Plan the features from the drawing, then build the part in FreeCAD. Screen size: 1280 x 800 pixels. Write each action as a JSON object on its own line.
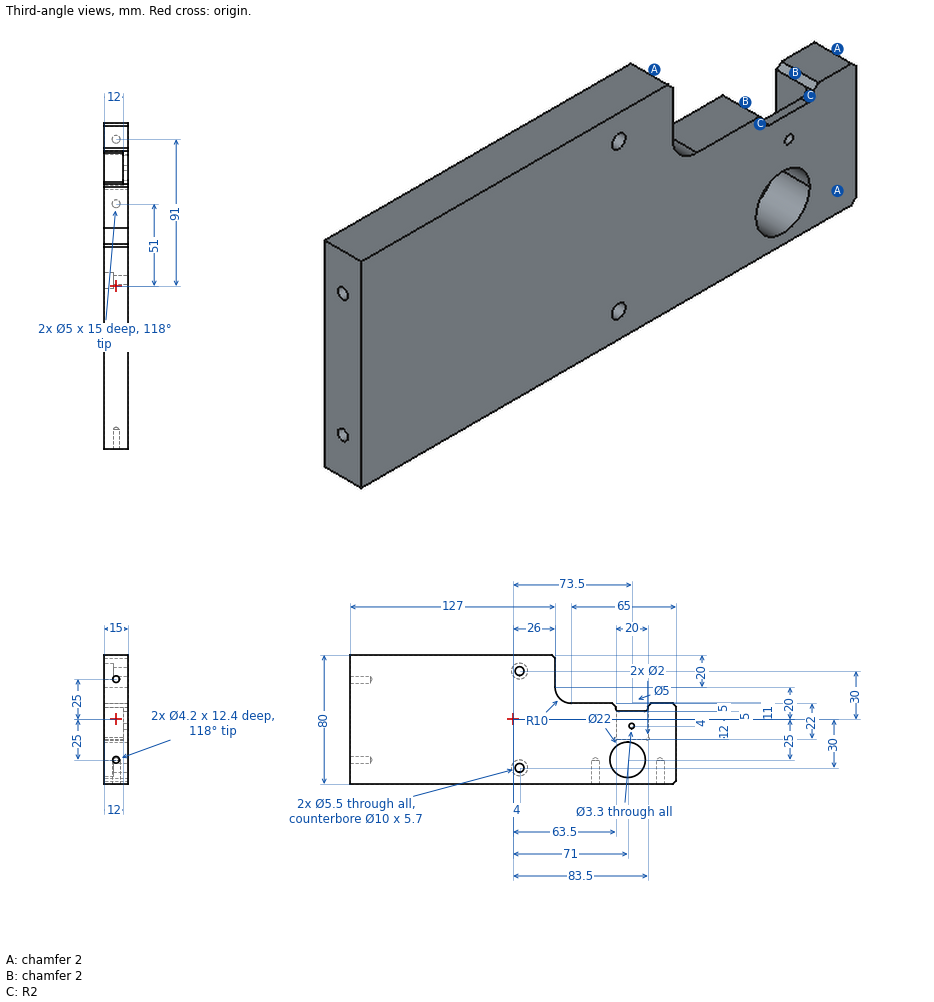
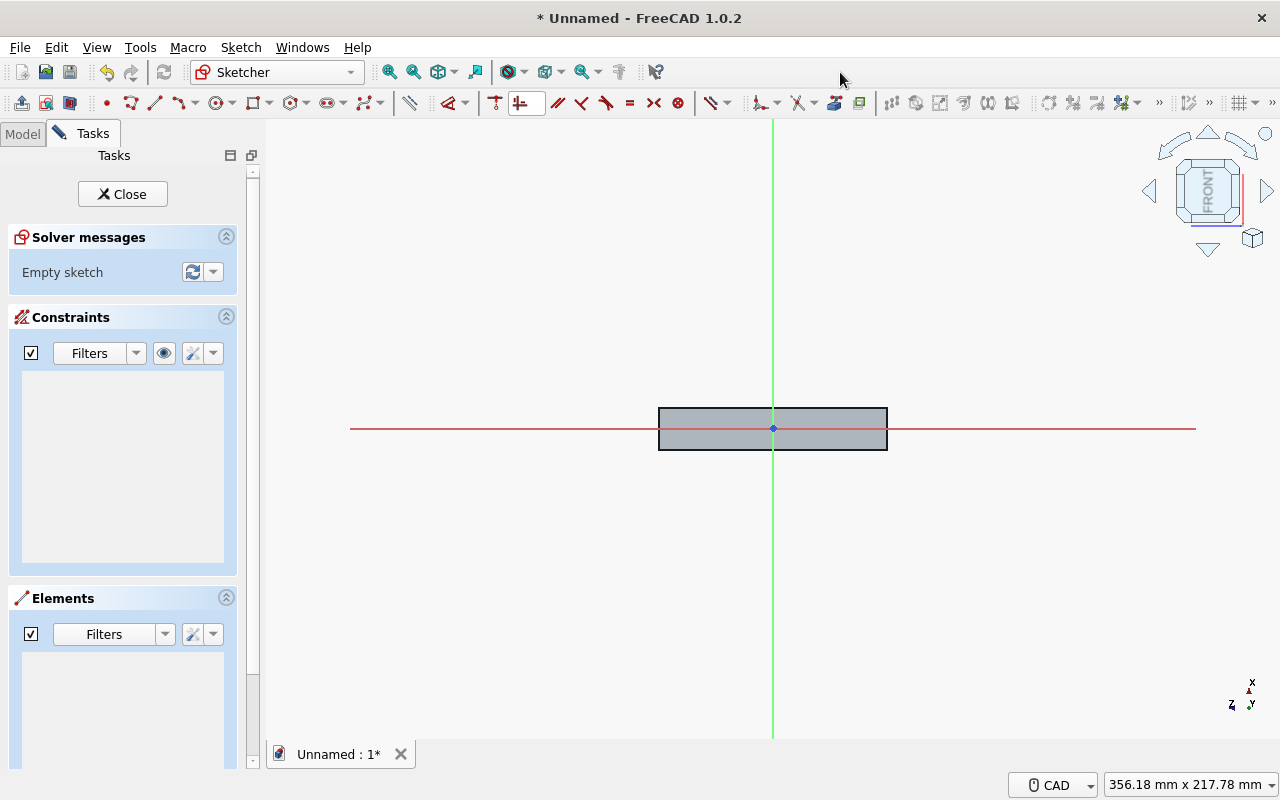
{"action": "scroll", "coordinate": [795, 429], "scroll_direction": "up", "scroll_amount": 7}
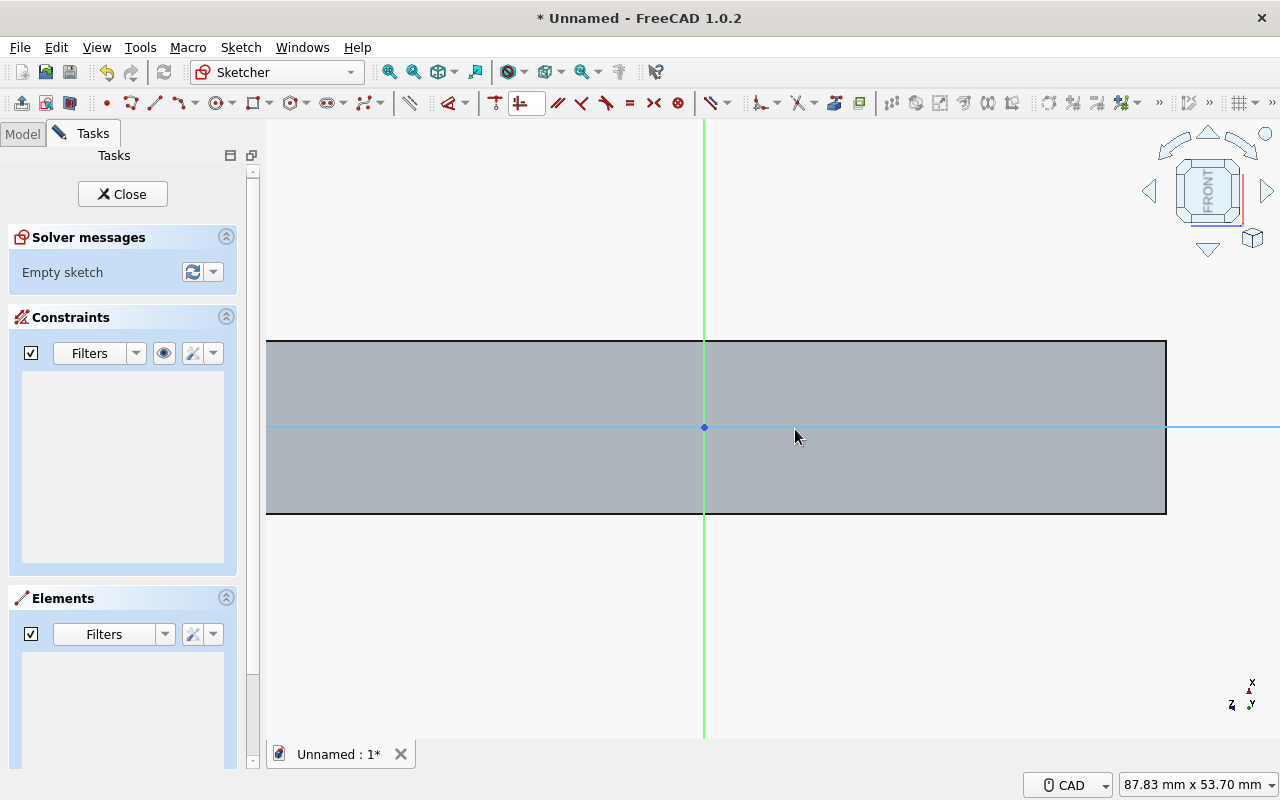
{"action": "left_click", "coordinate": [216, 104]}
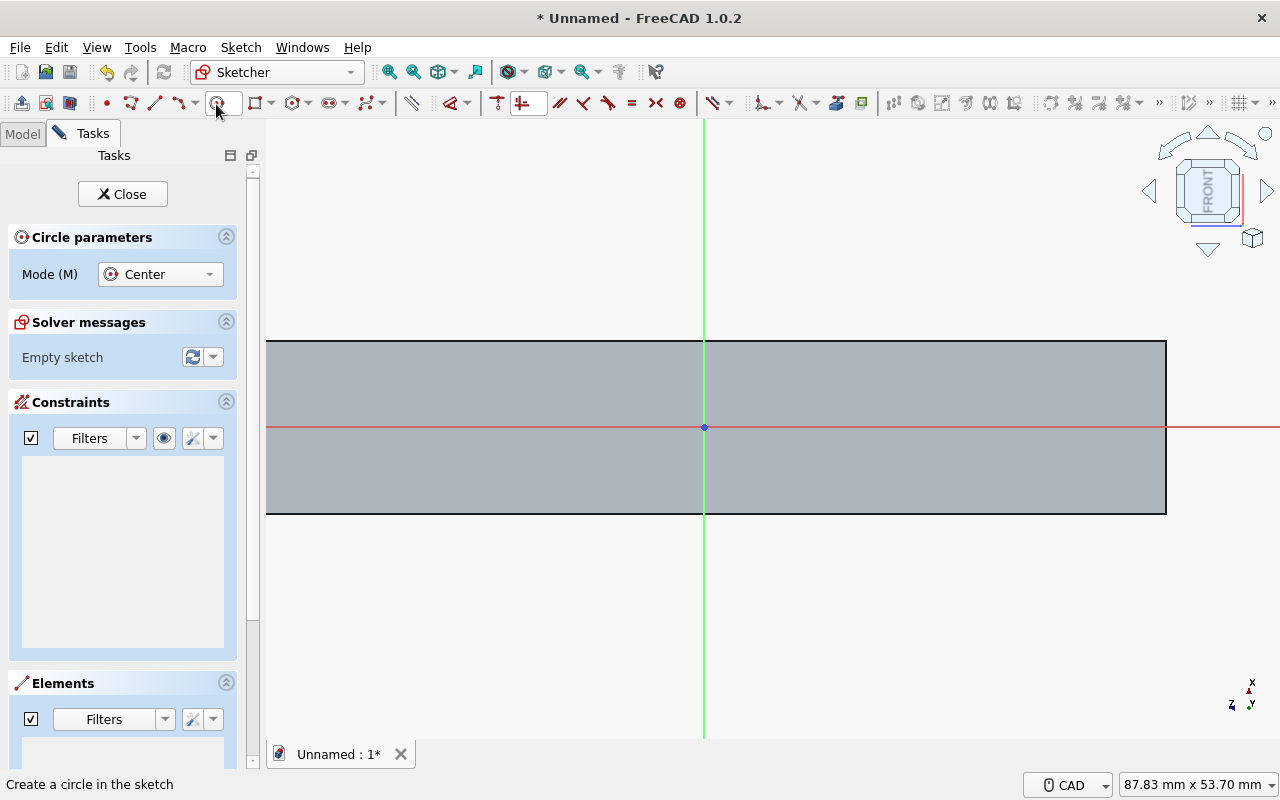
{"action": "left_click", "coordinate": [993, 427]}
{"action": "left_click", "coordinate": [1010, 410]}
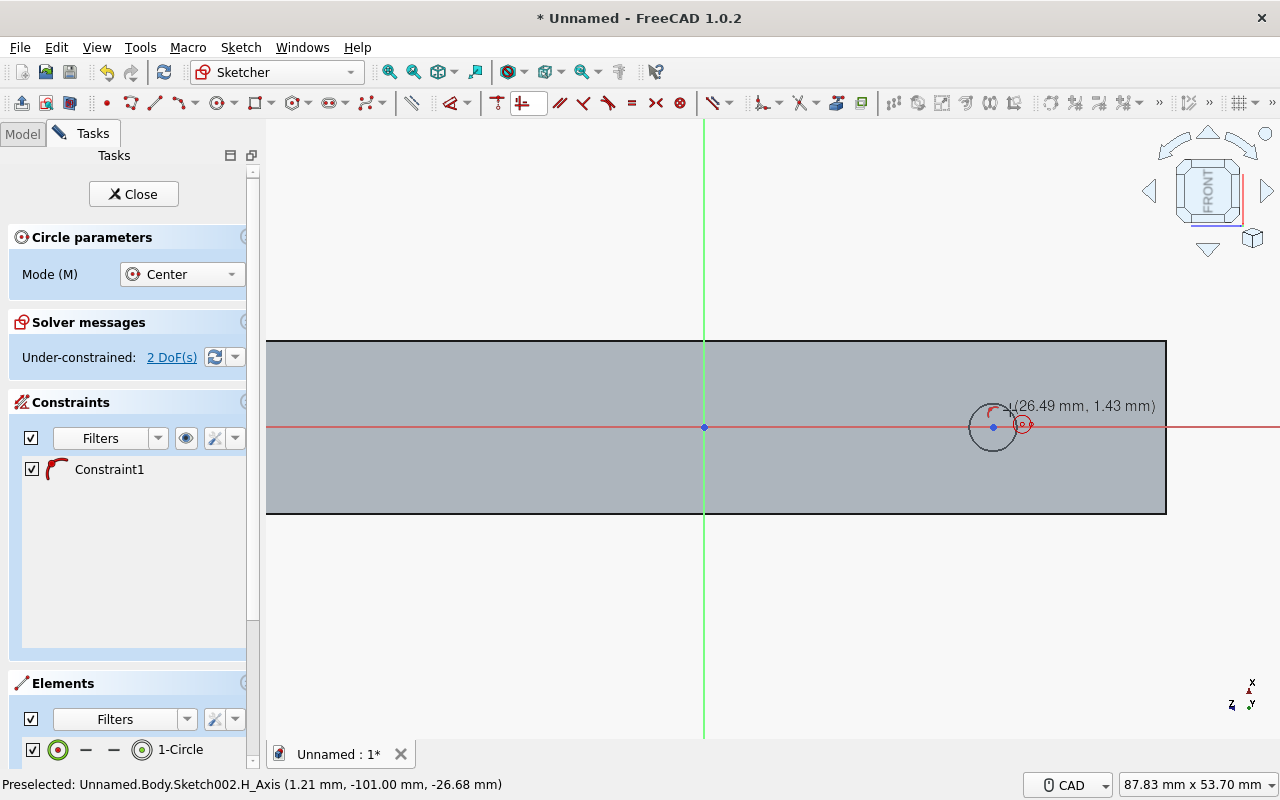
{"action": "left_click", "coordinate": [416, 427]}
{"action": "left_click", "coordinate": [433, 410]}
{"action": "key", "text": "Escape"}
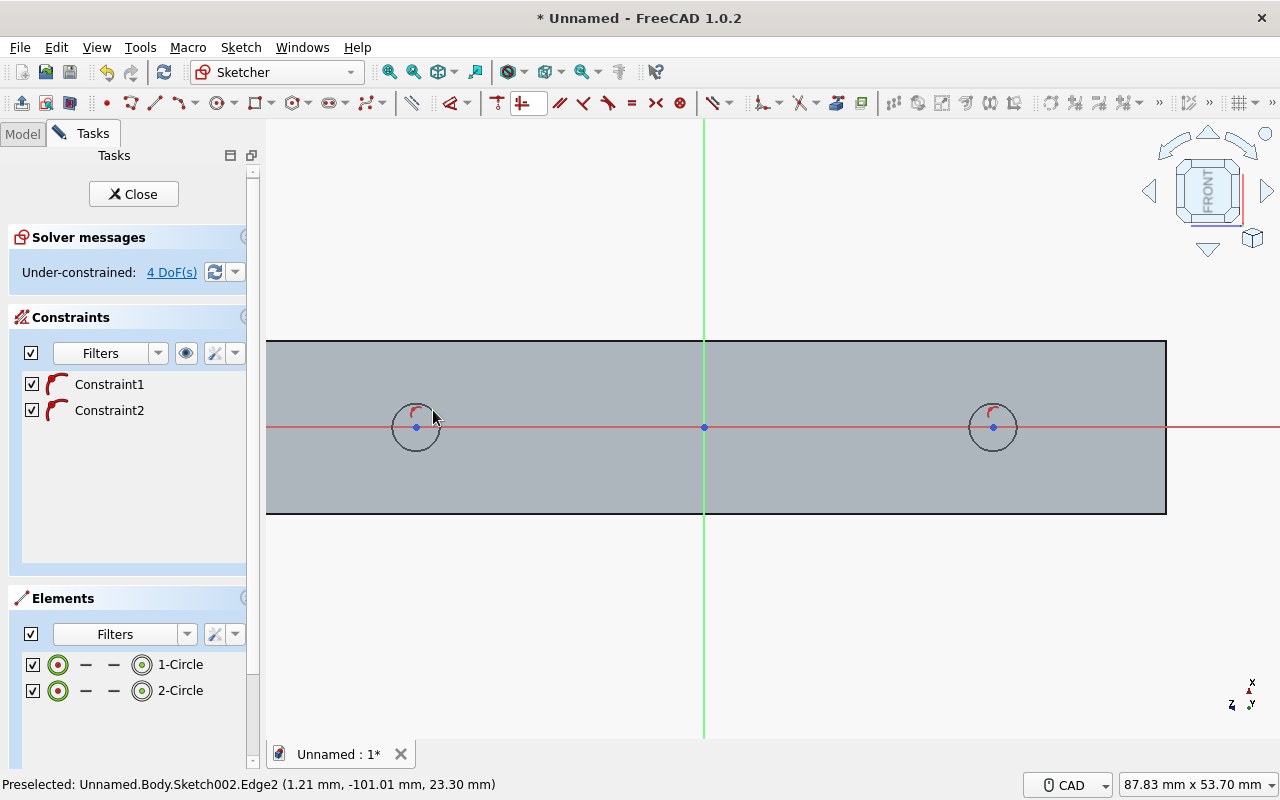
{"action": "left_click", "coordinate": [1010, 411]}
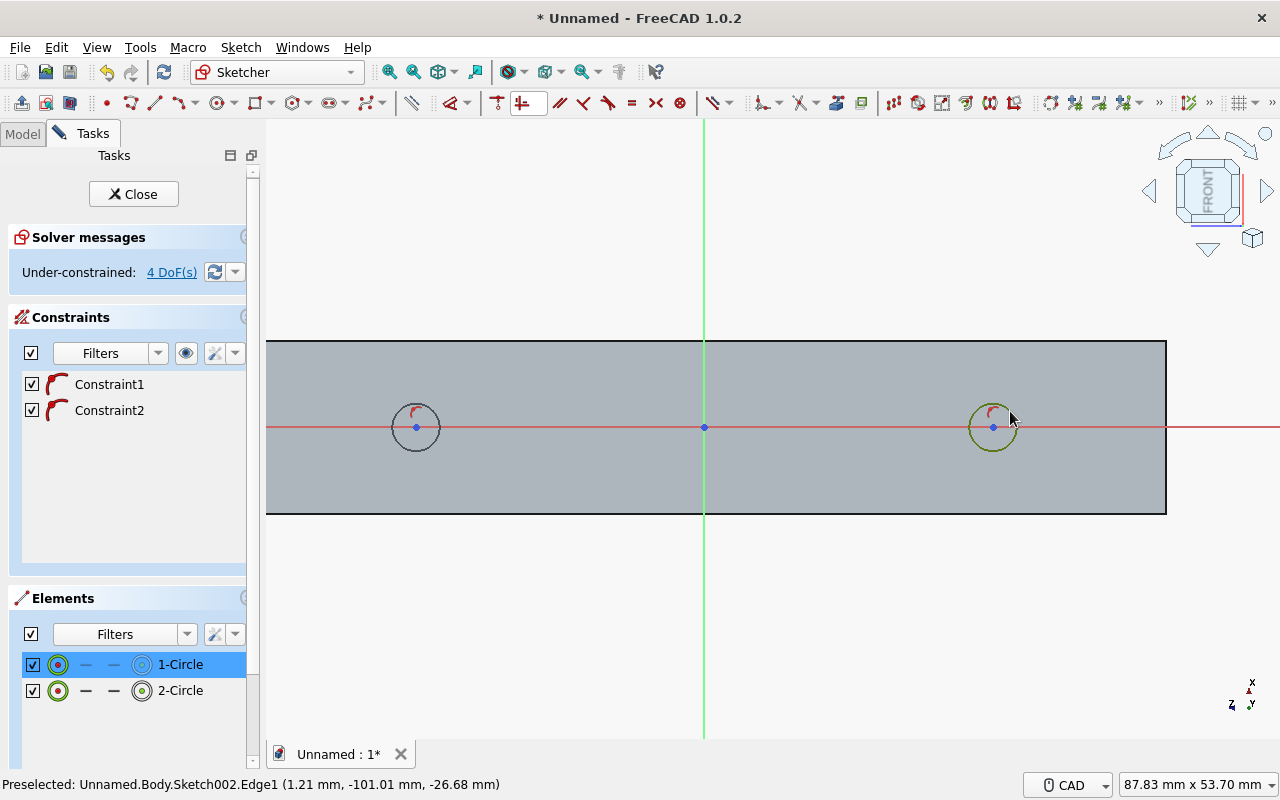
{"action": "left_click", "coordinate": [433, 411]}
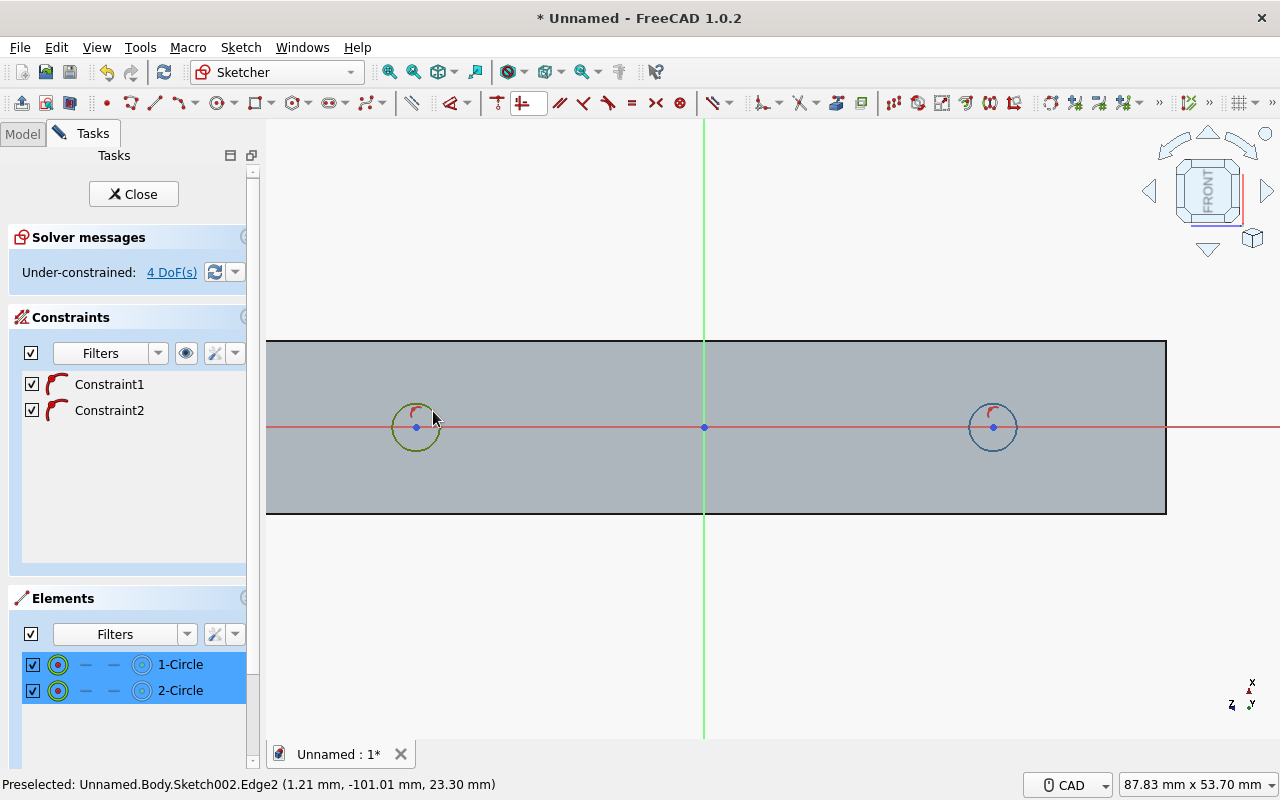
{"action": "left_click", "coordinate": [632, 104]}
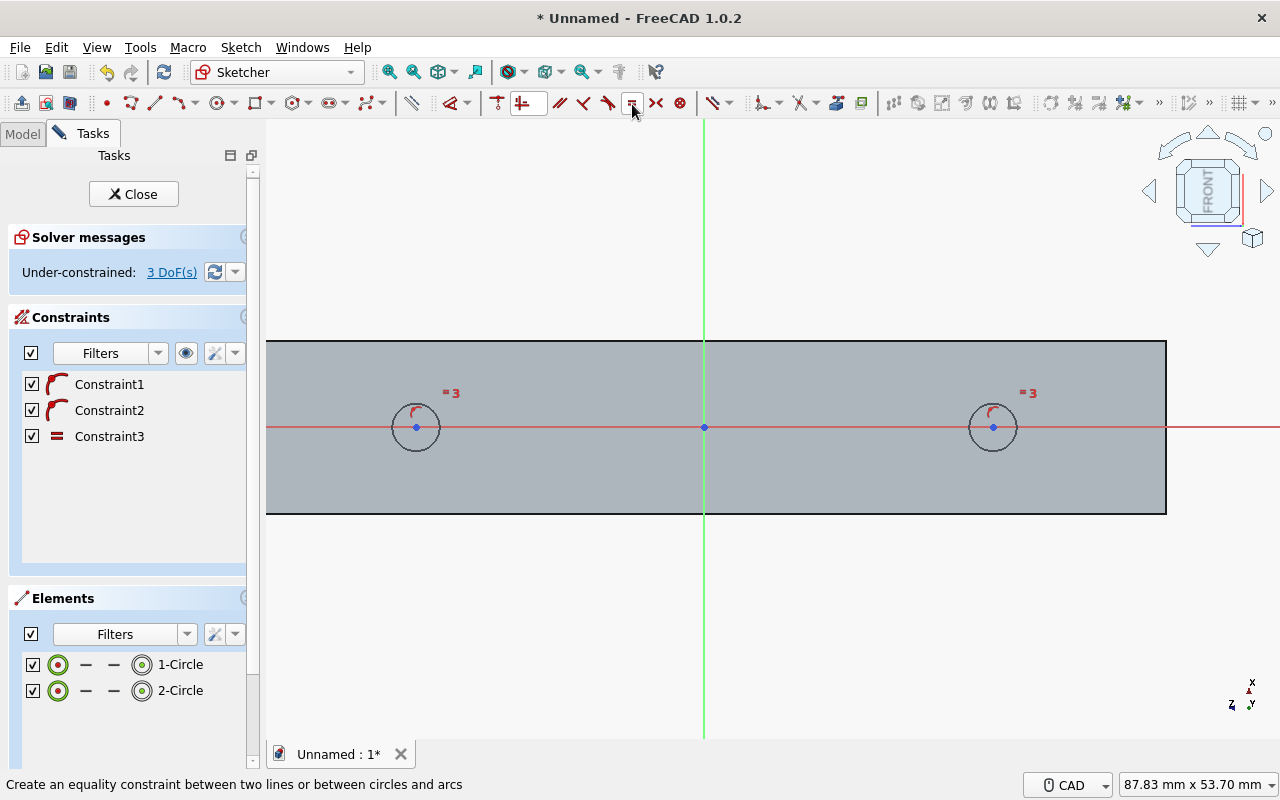
{"action": "left_click", "coordinate": [450, 104]}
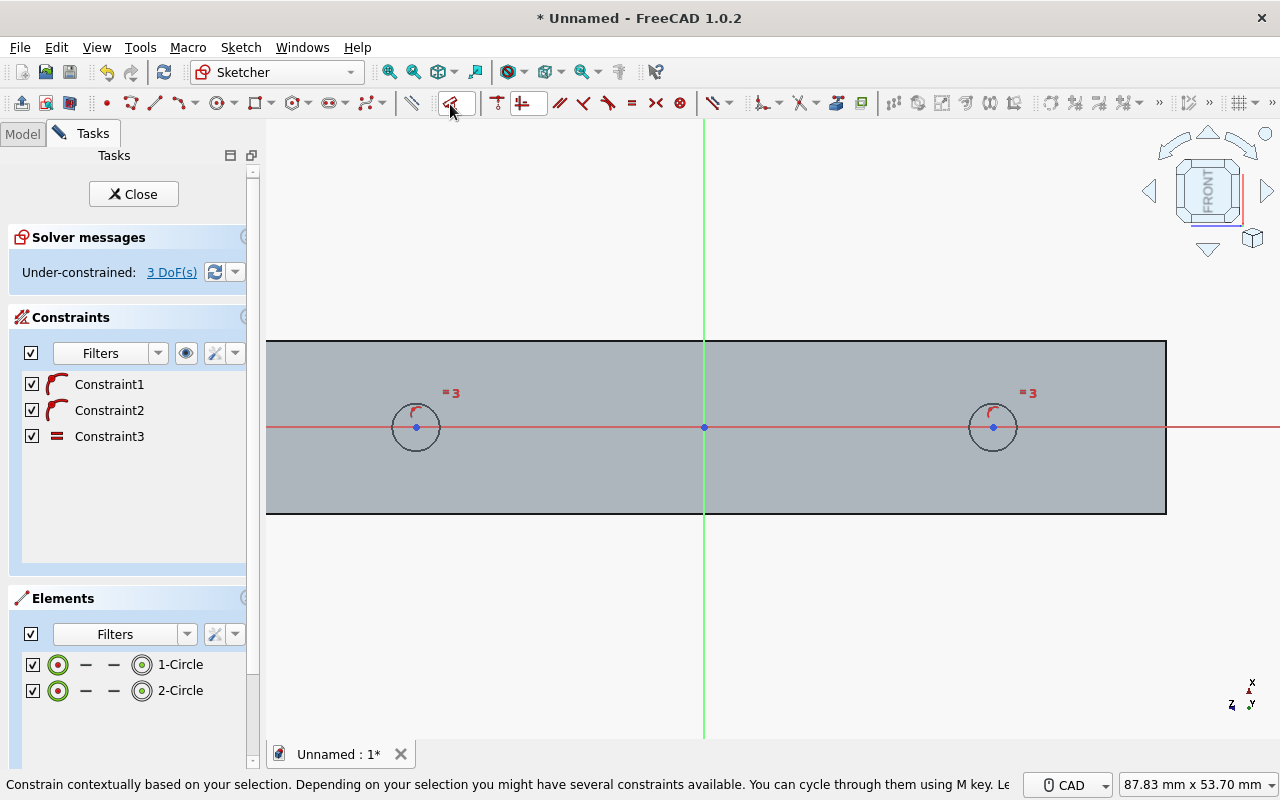
{"action": "left_click", "coordinate": [1010, 411]}
{"action": "left_click", "coordinate": [1033, 389]}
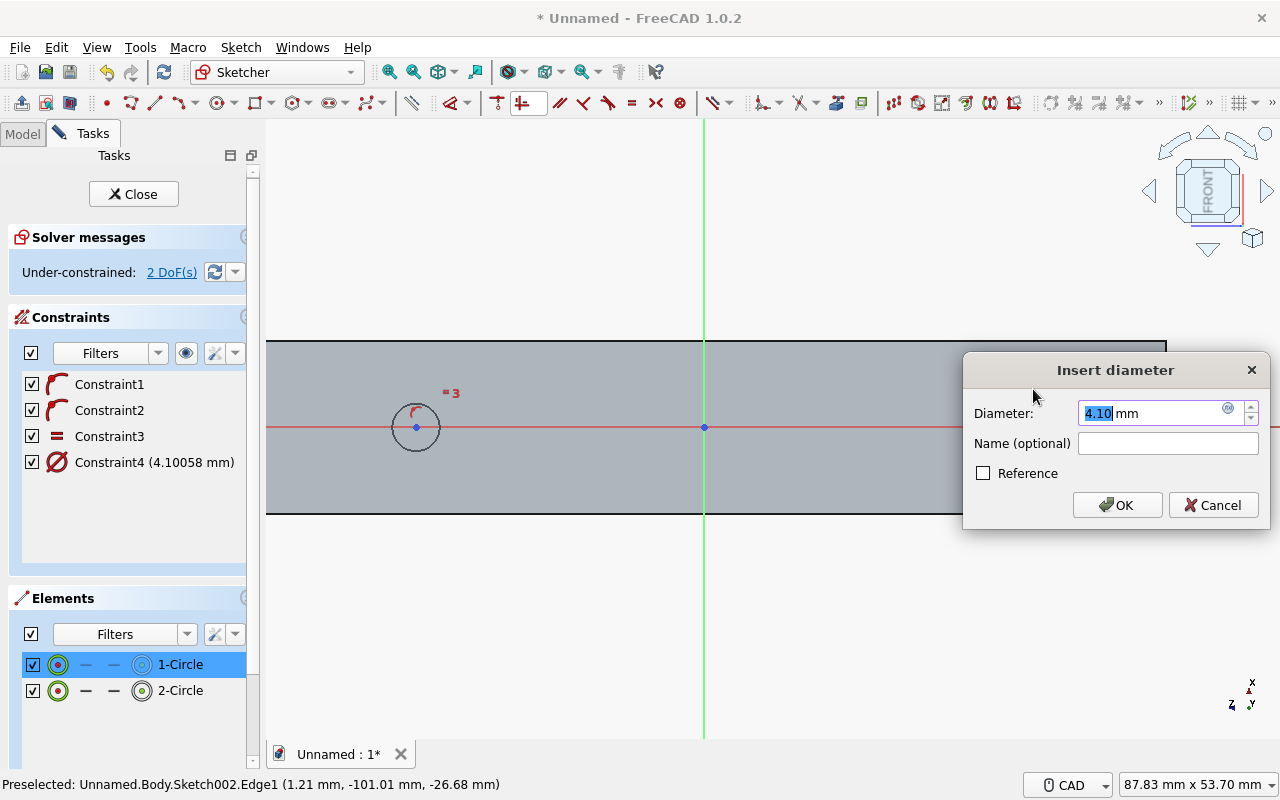
{"action": "type", "text": "4.2"}
{"action": "key", "text": "Return"}